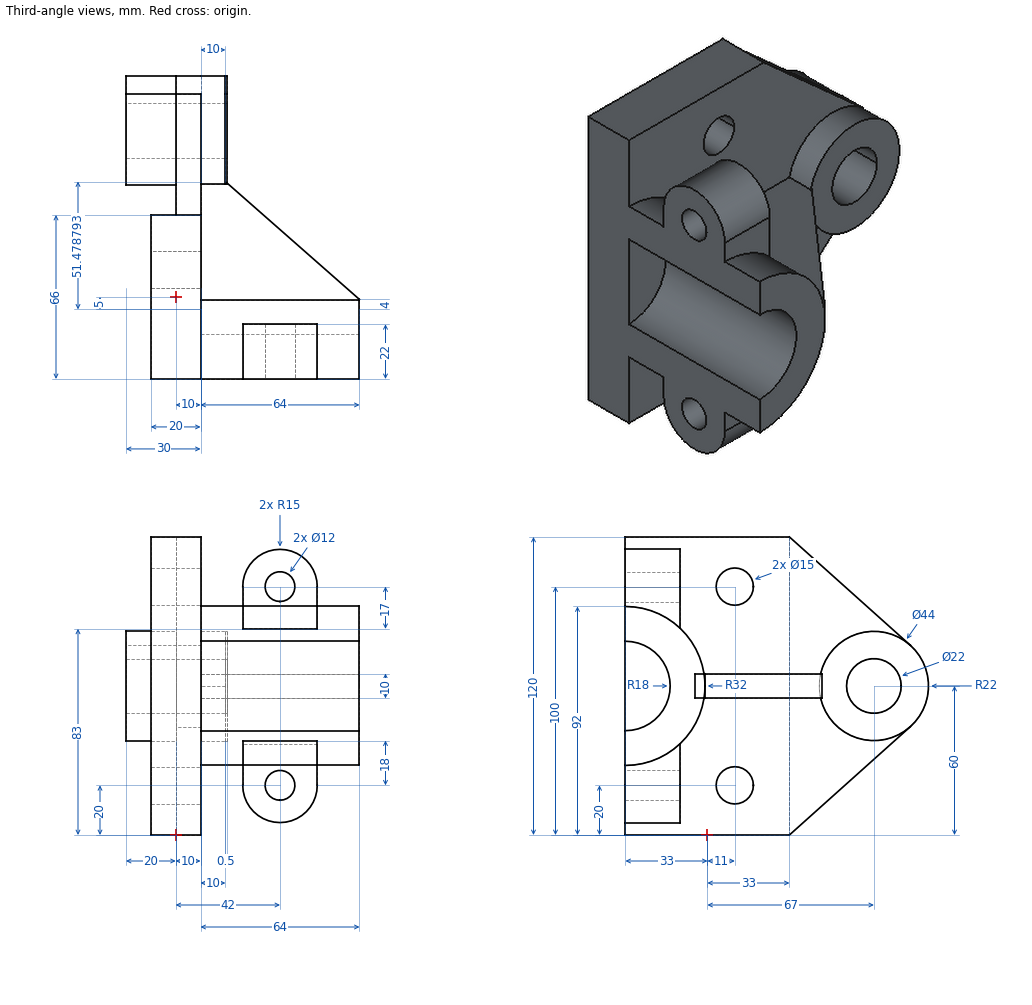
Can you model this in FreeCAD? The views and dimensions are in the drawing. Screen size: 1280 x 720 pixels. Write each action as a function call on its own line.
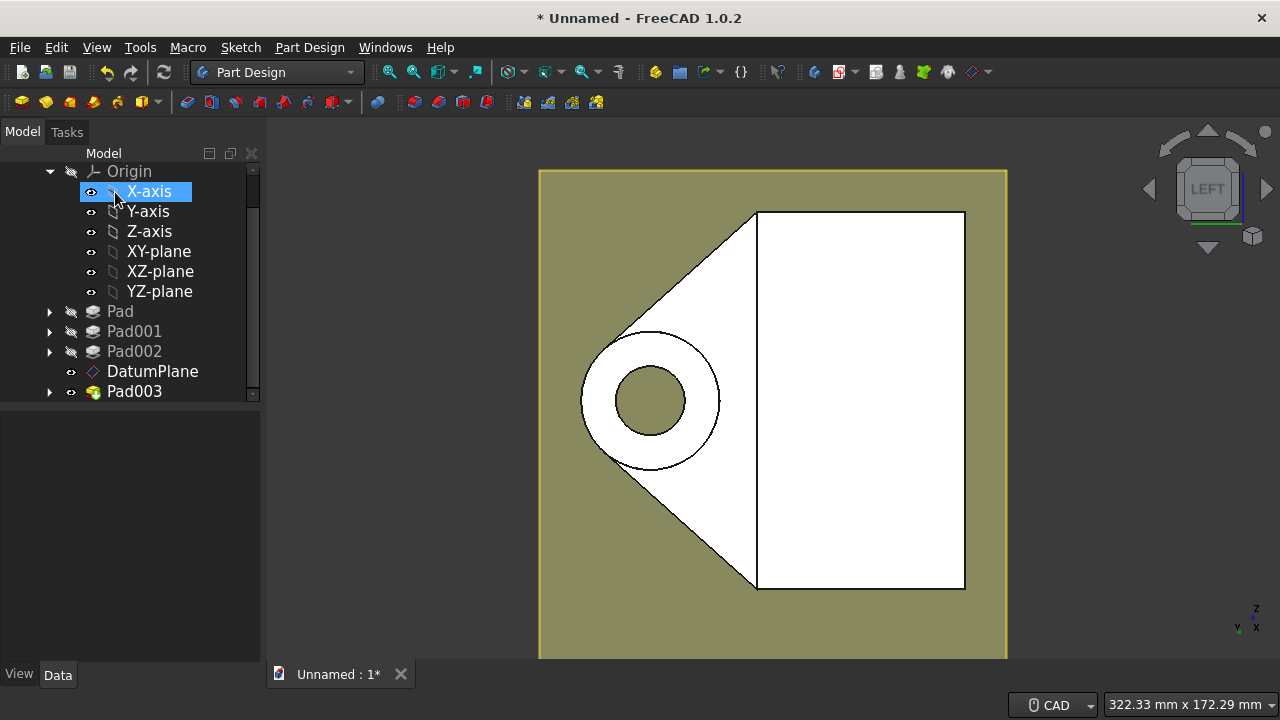
click(116, 372)
key(space)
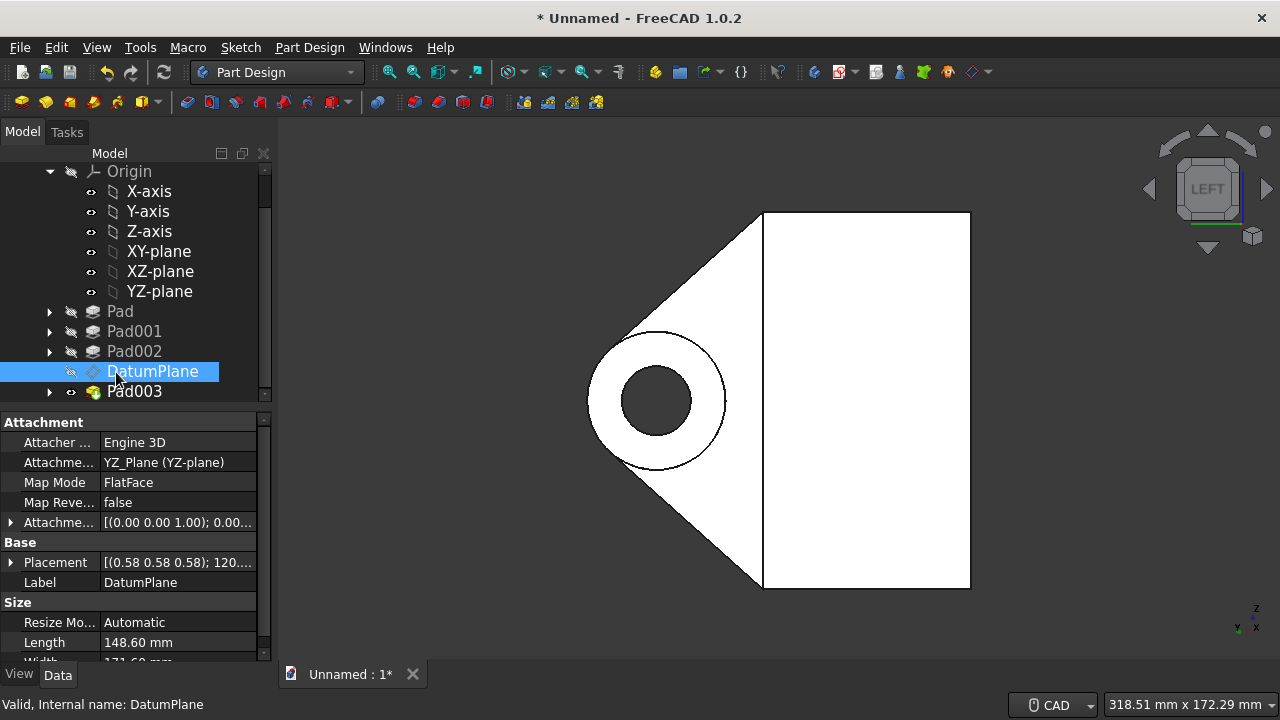
key(0)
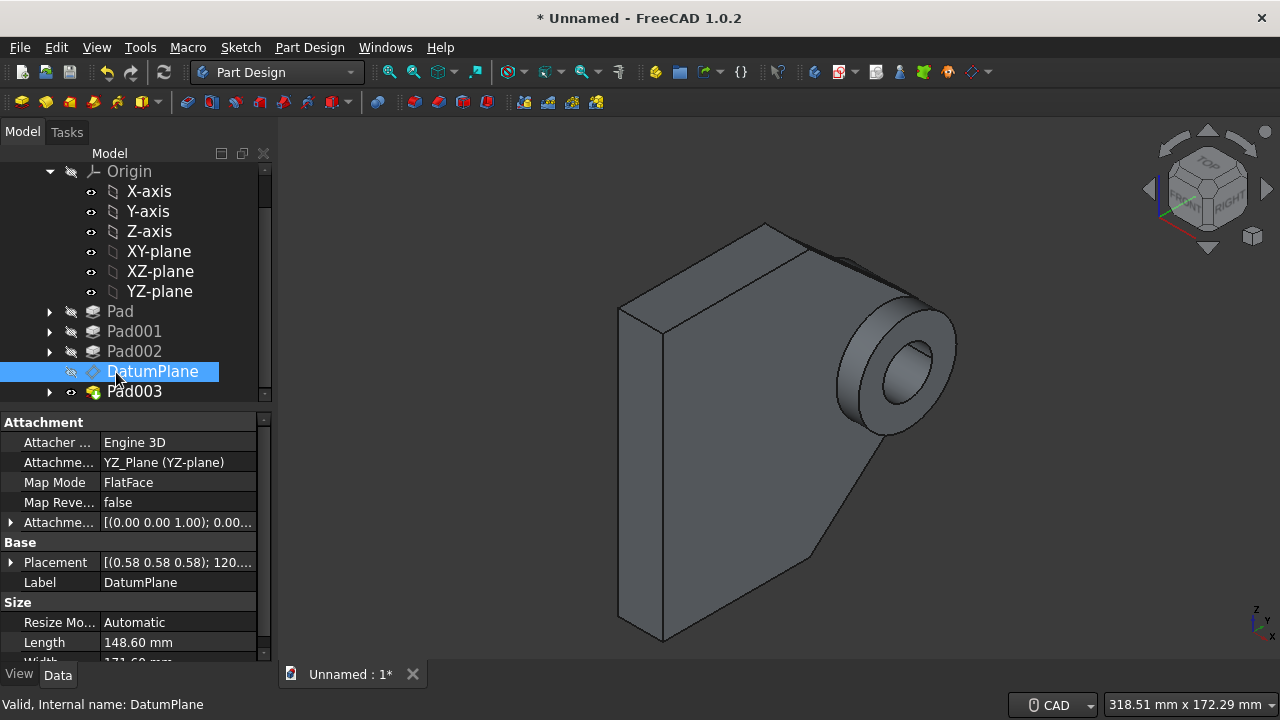
click(754, 478)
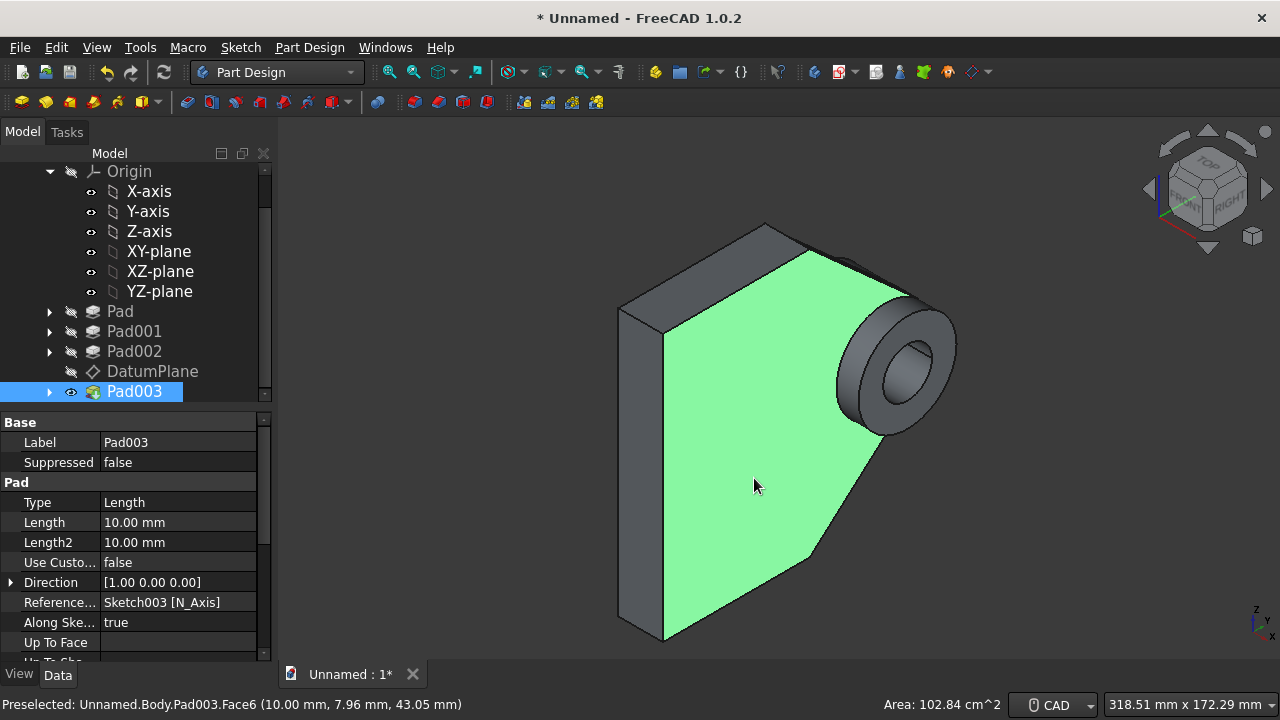
click(840, 72)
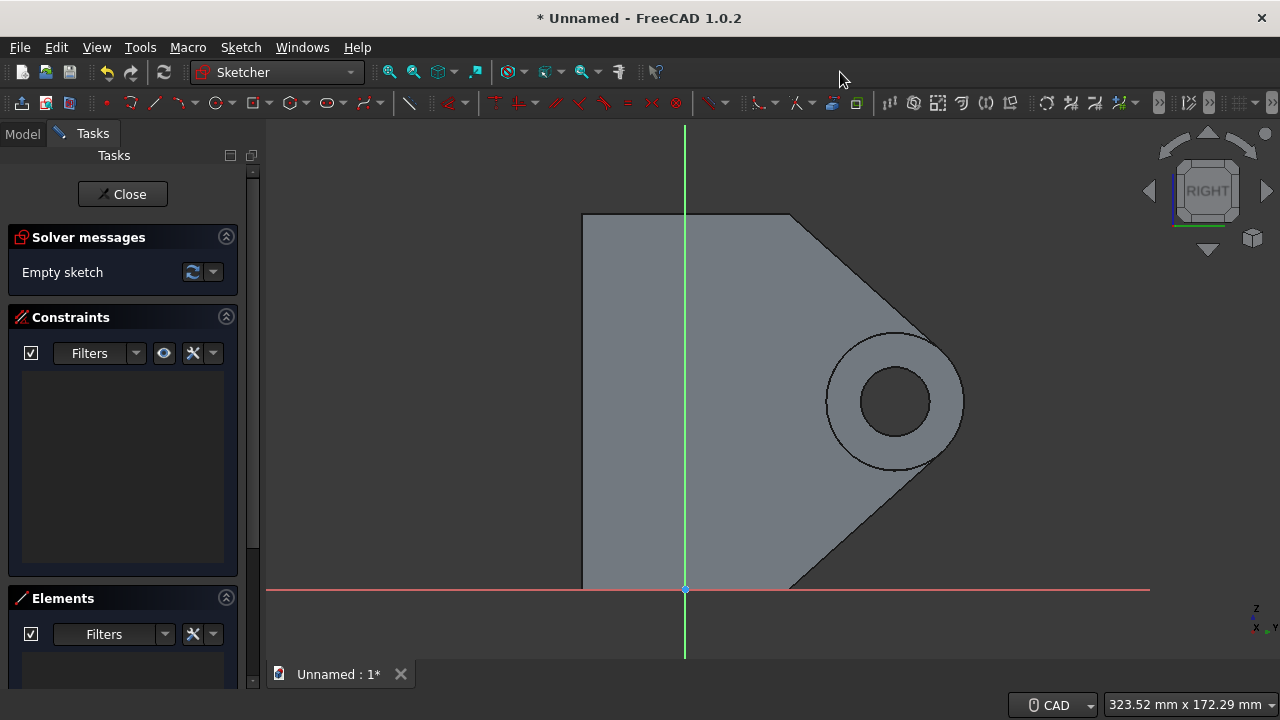
click(70, 104)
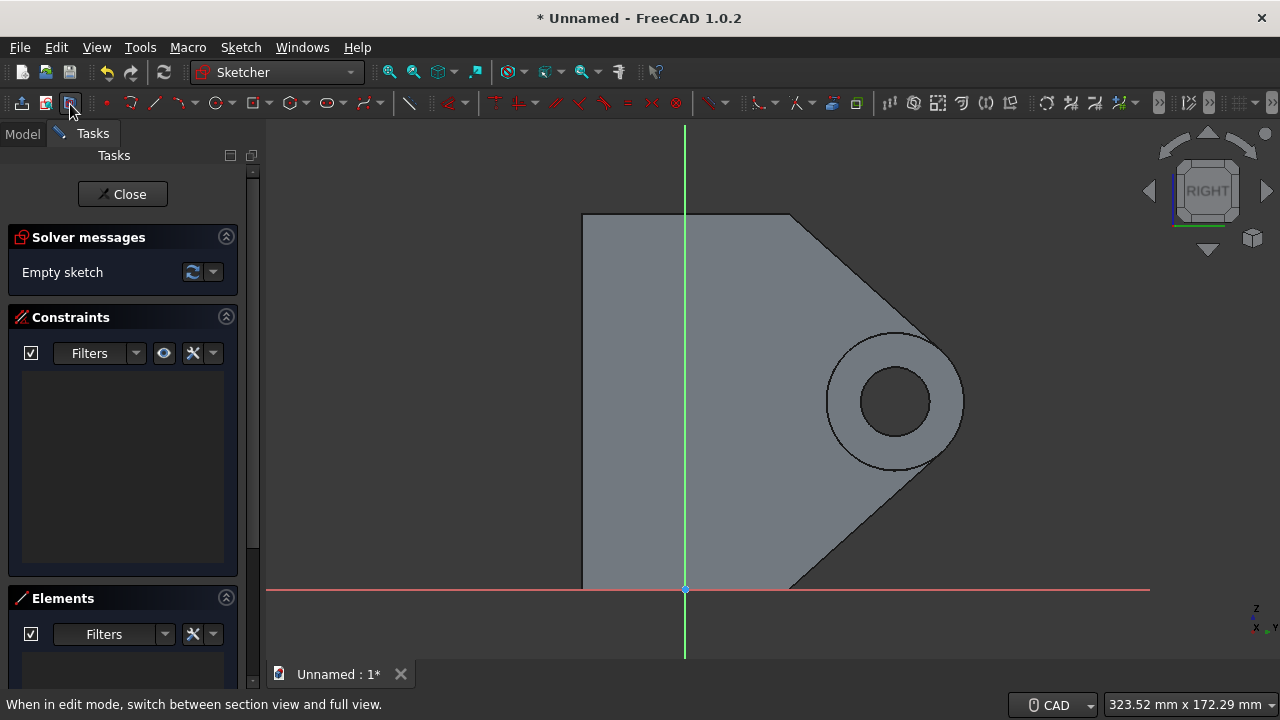
click(216, 104)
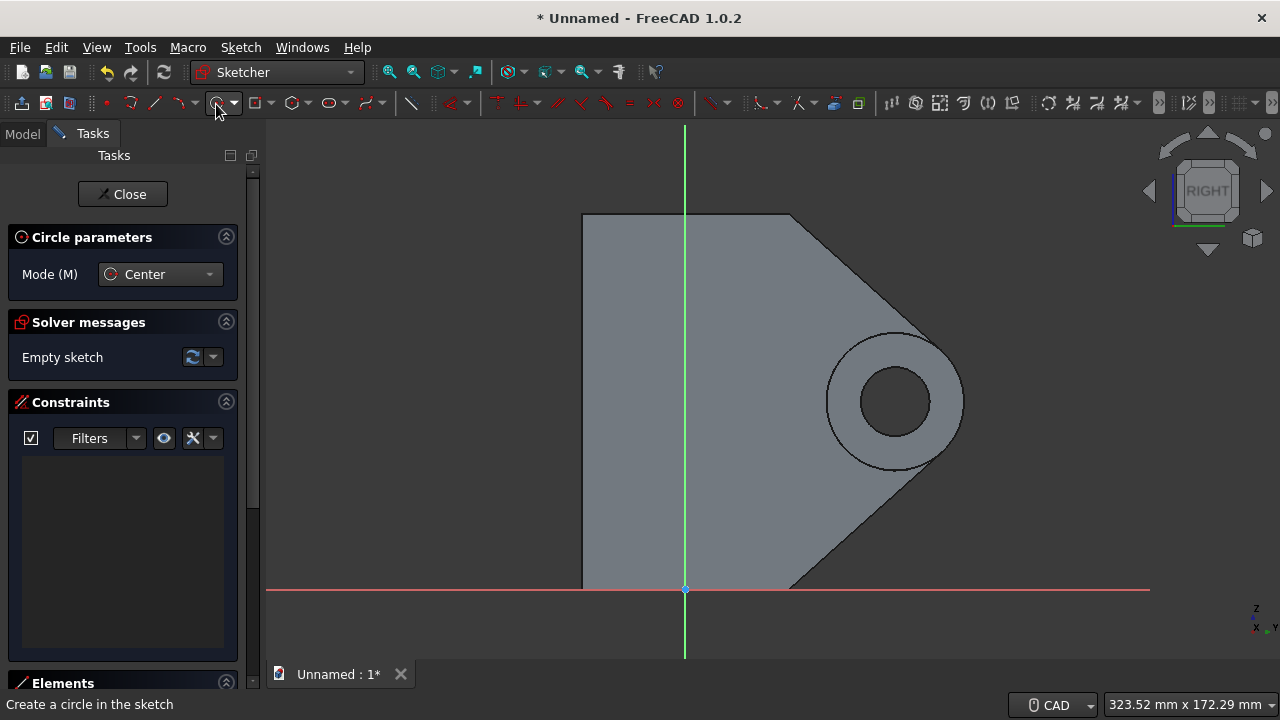
click(720, 276)
click(736, 260)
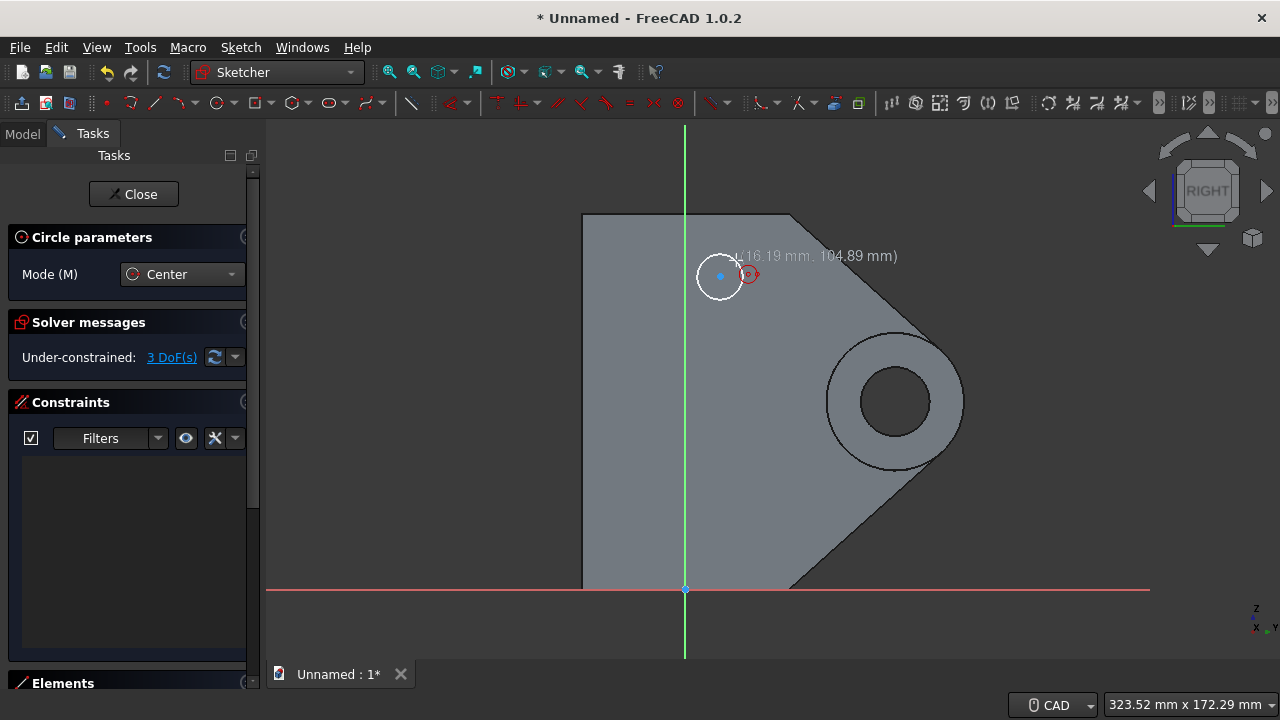
click(720, 527)
click(736, 510)
key(Escape)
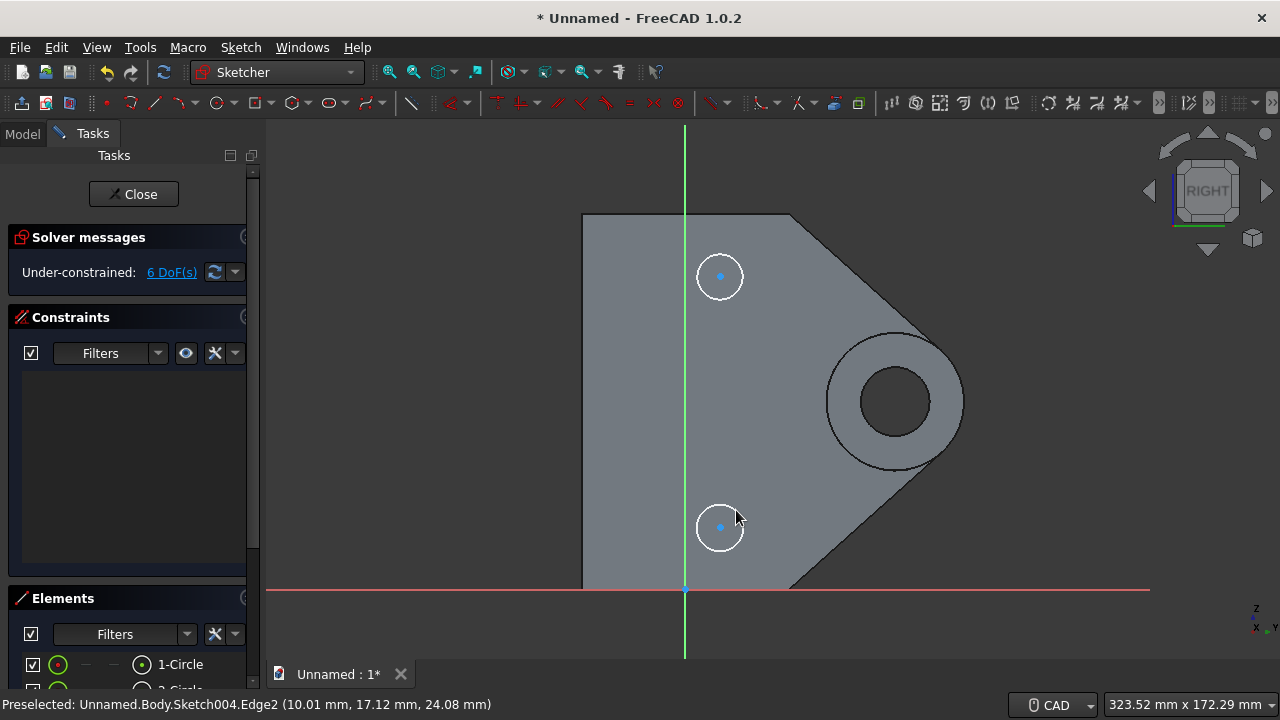
click(736, 261)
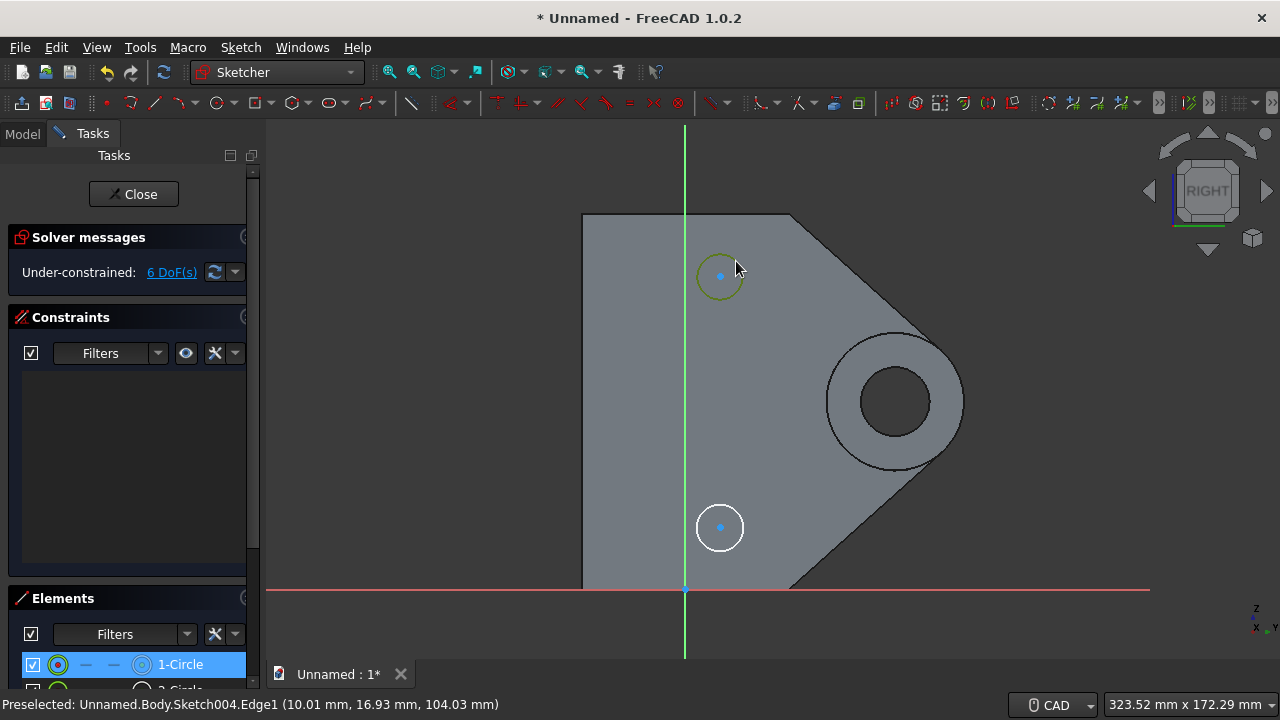
click(736, 511)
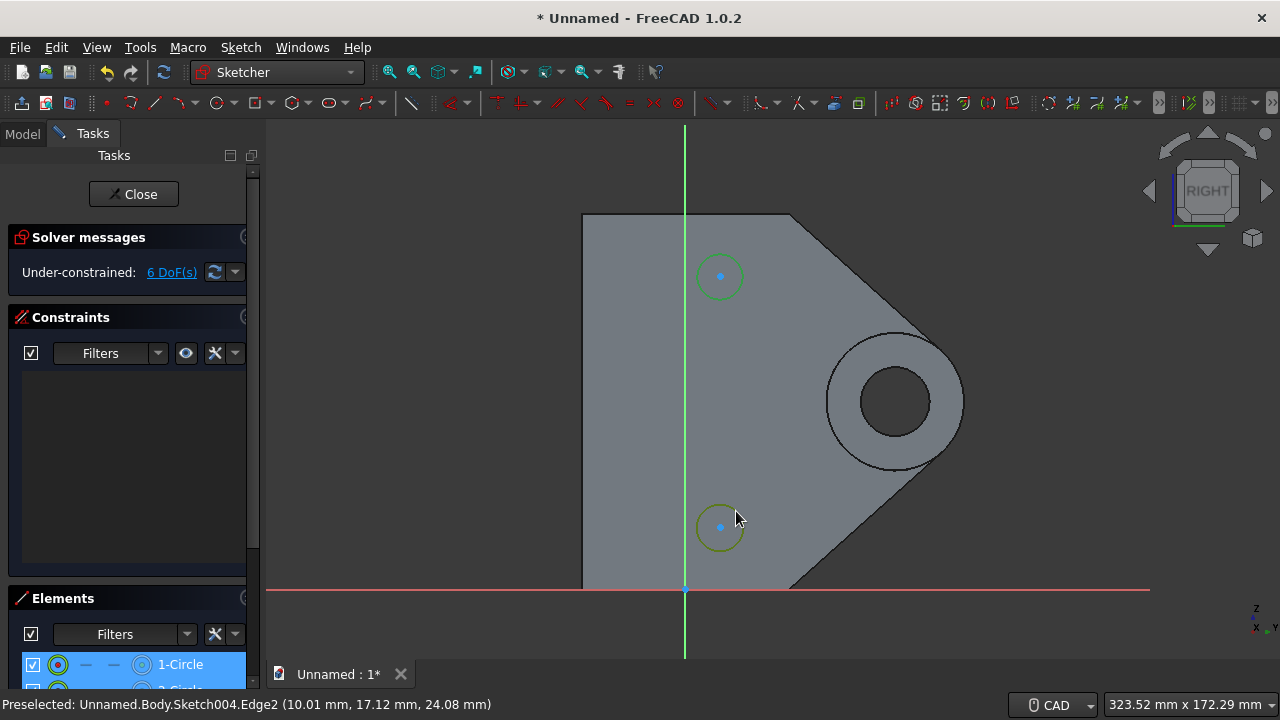
click(630, 104)